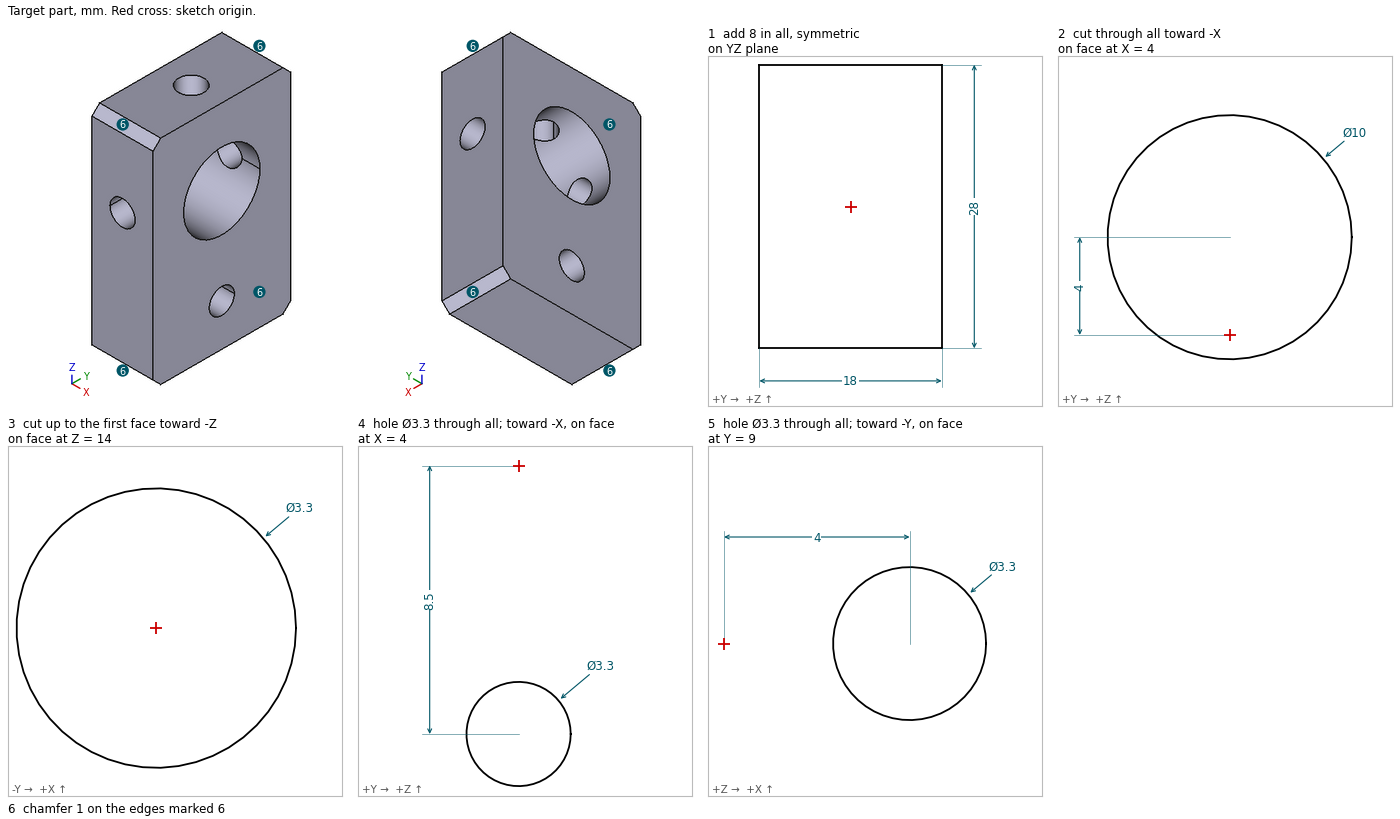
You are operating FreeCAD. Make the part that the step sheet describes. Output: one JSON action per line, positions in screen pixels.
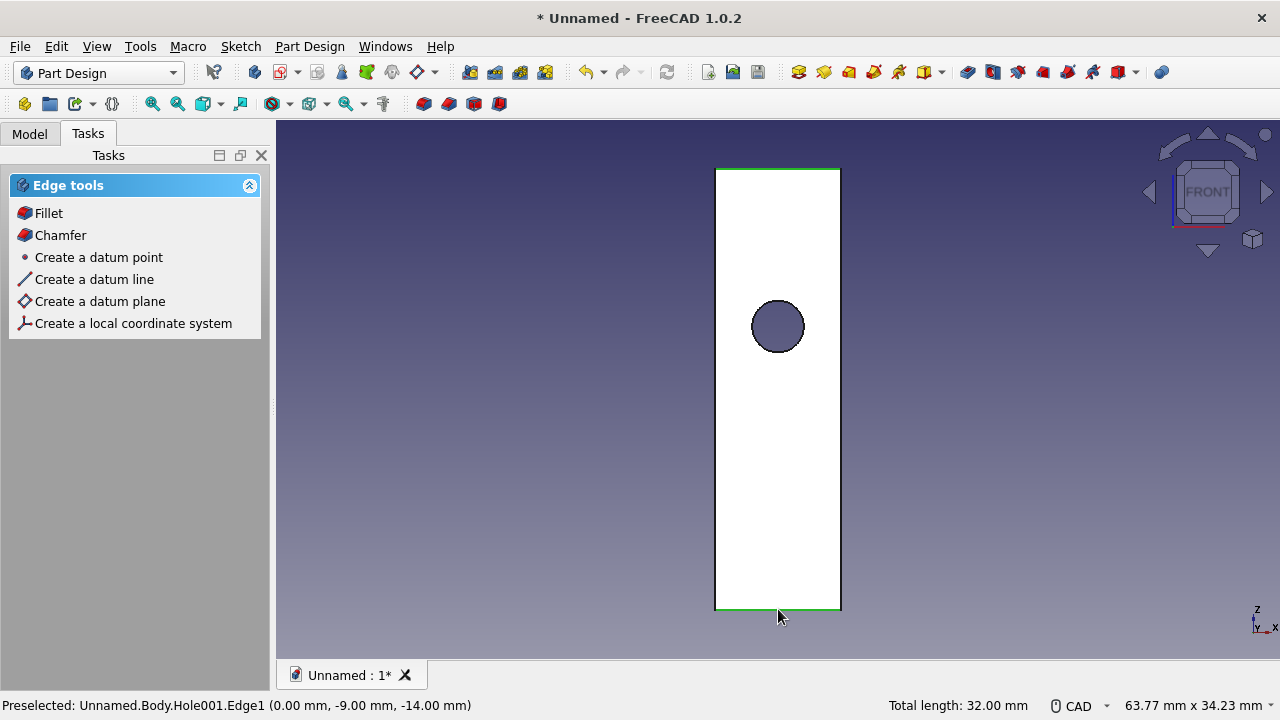
{"action": "left_click", "coordinate": [449, 104]}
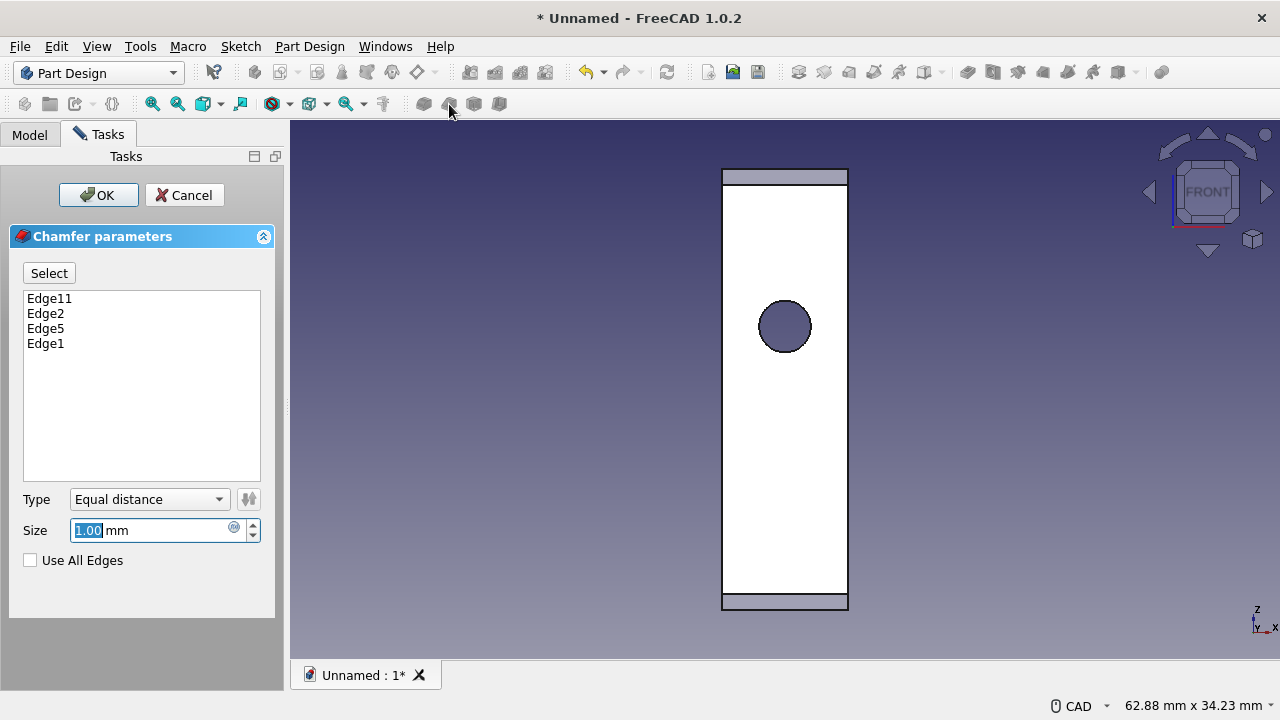
{"action": "type", "text": "1"}
{"action": "key", "text": "Tab"}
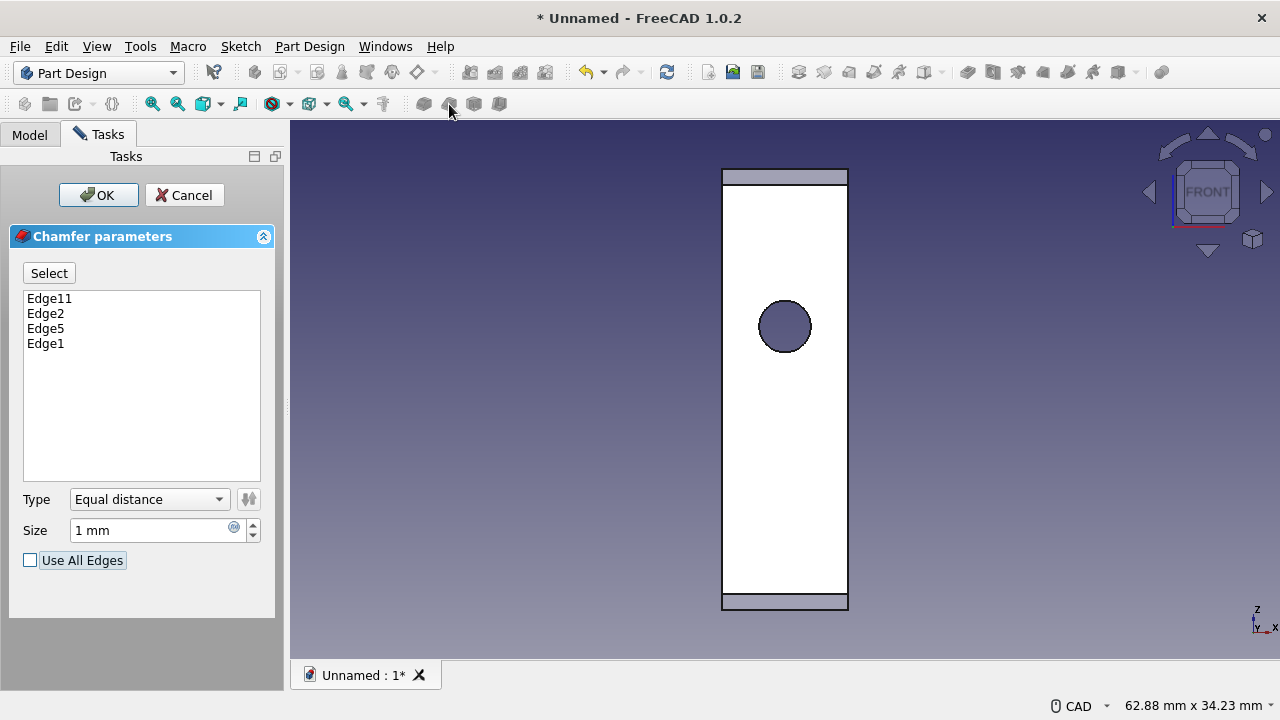
{"action": "left_click", "coordinate": [99, 195]}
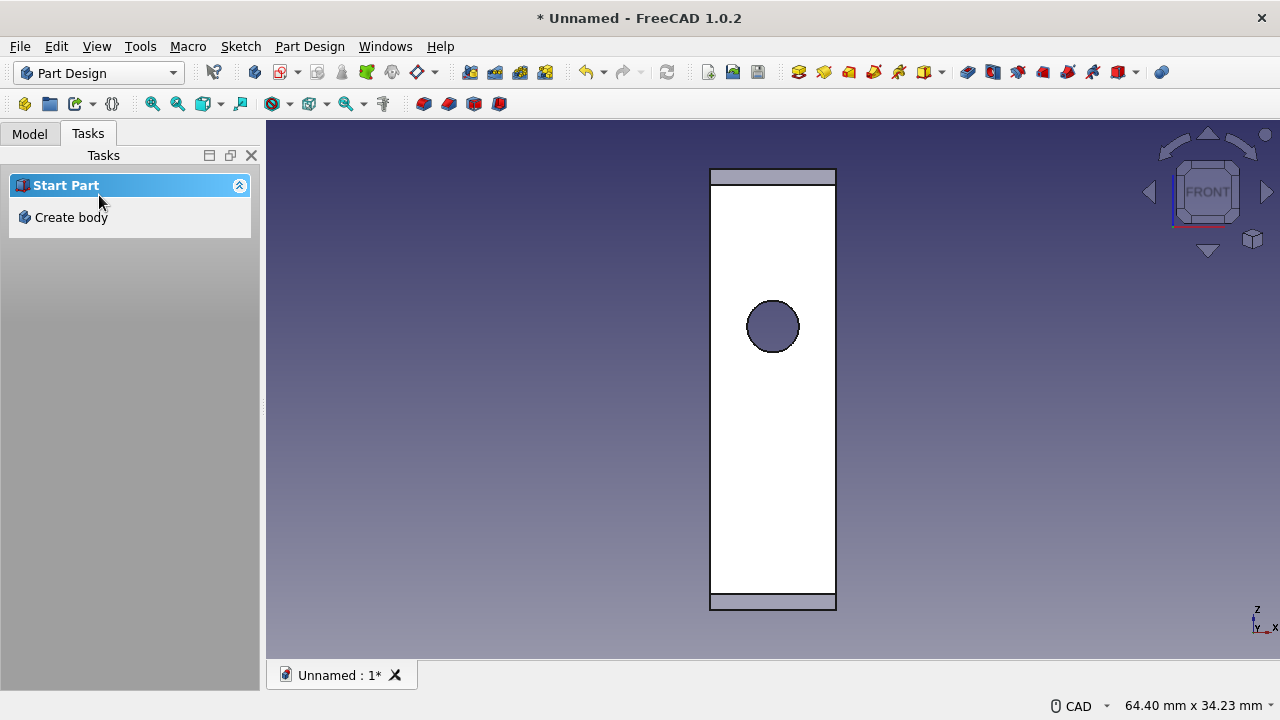
{"action": "key", "text": "0"}